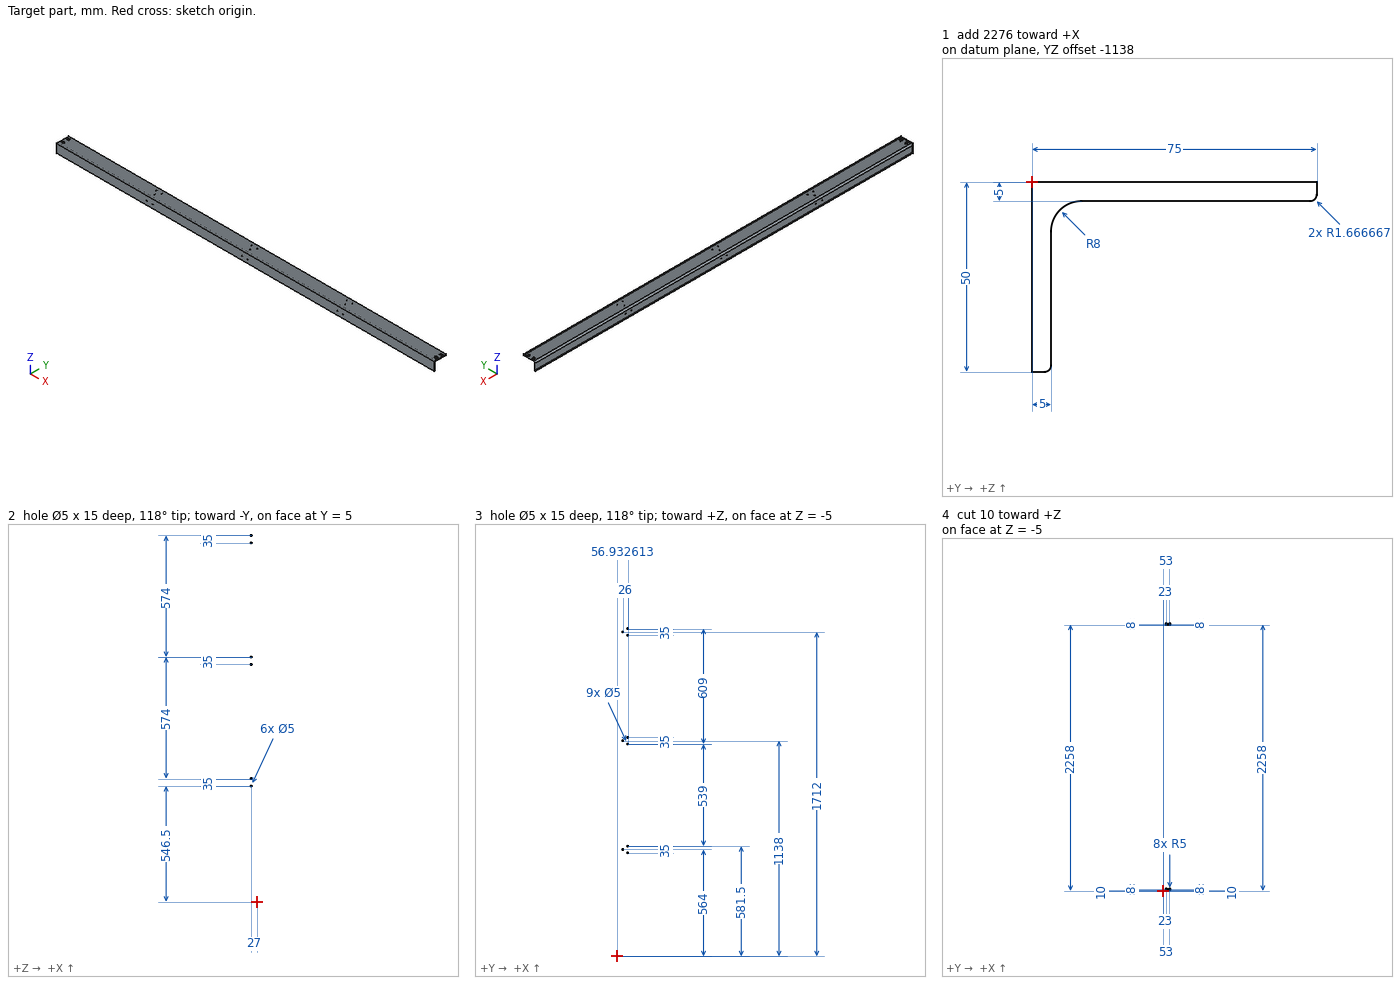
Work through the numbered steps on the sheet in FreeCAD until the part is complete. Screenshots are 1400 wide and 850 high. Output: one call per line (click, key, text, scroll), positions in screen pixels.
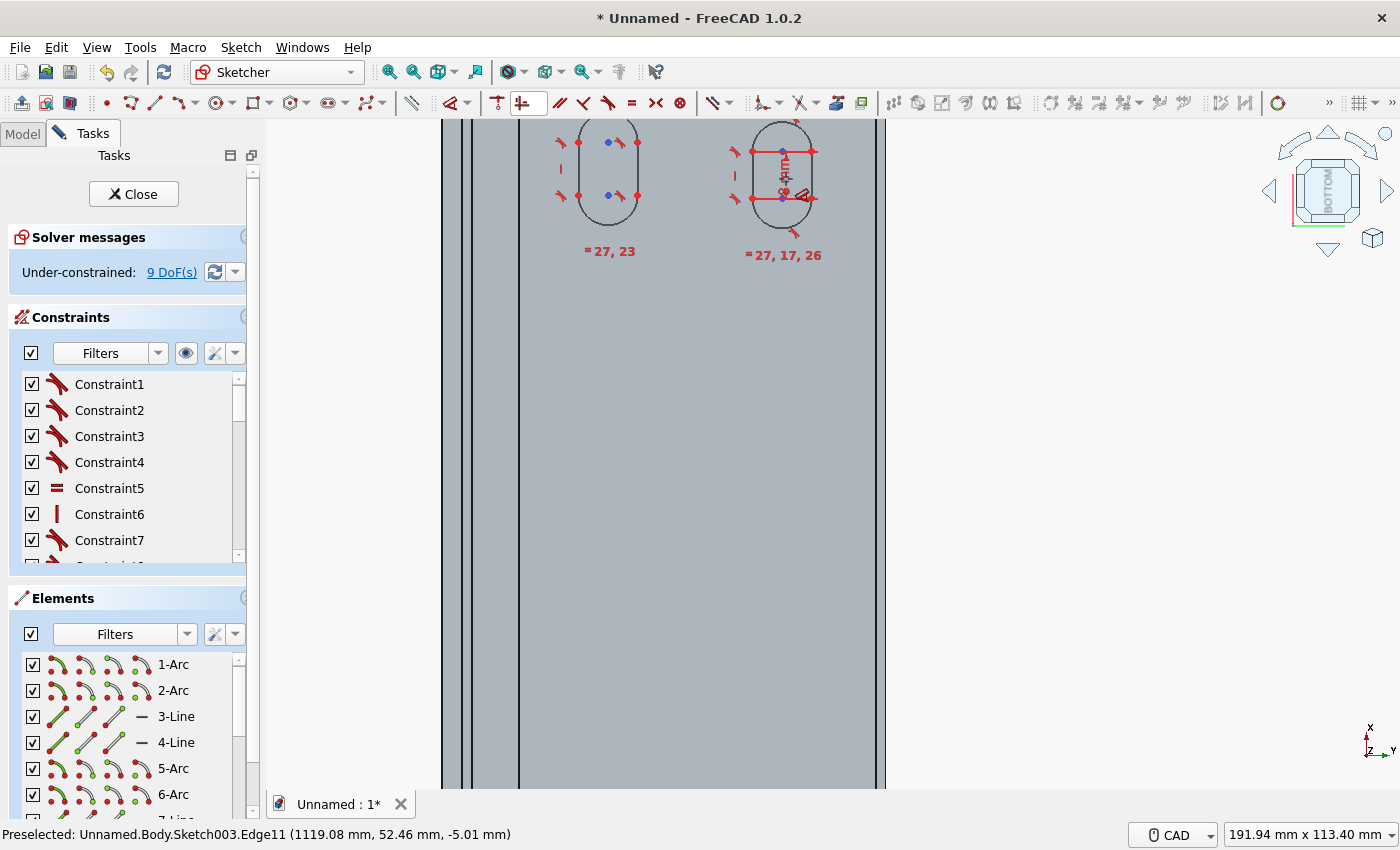
click(579, 179)
click(545, 171)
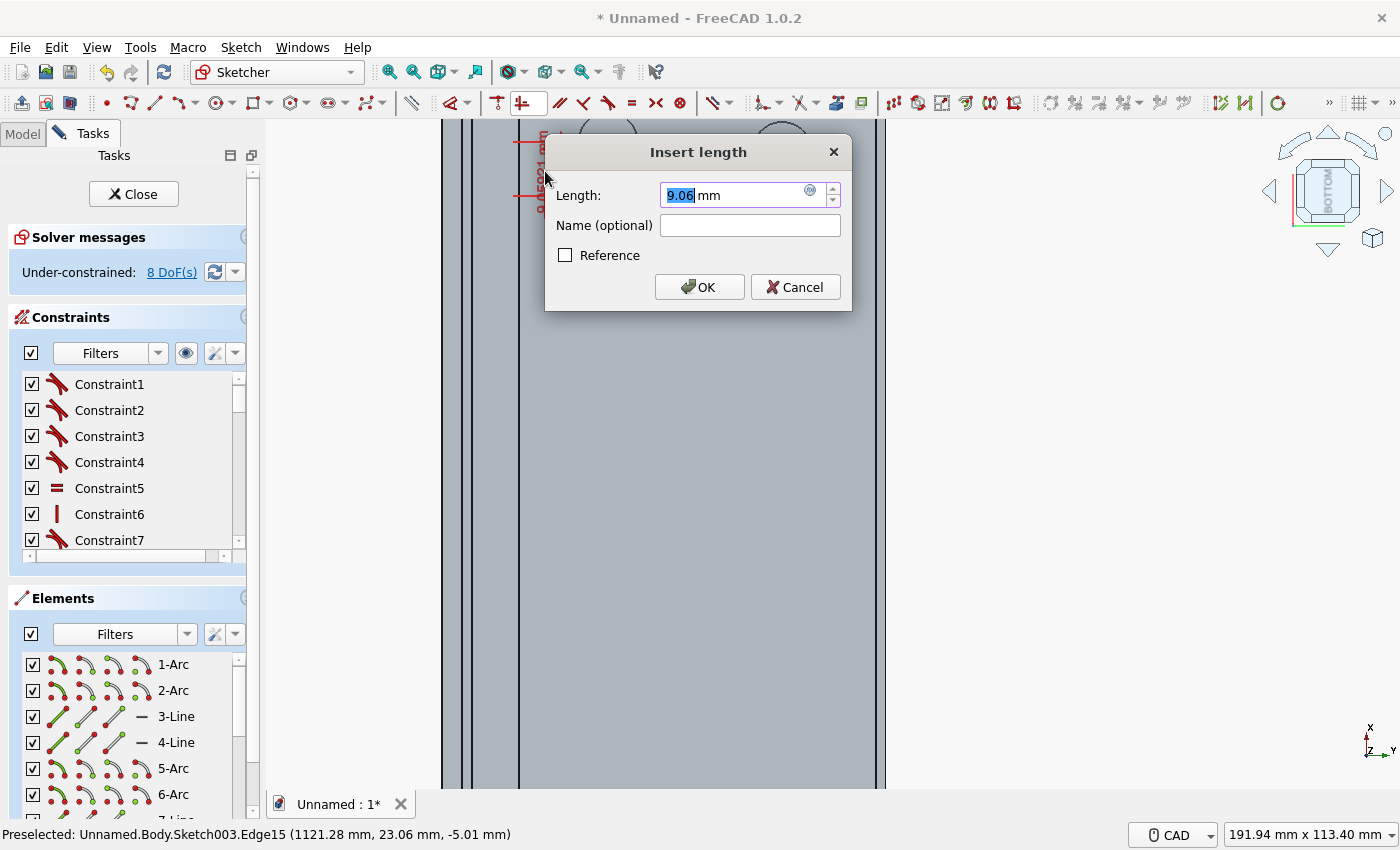
text(8)
key(Return)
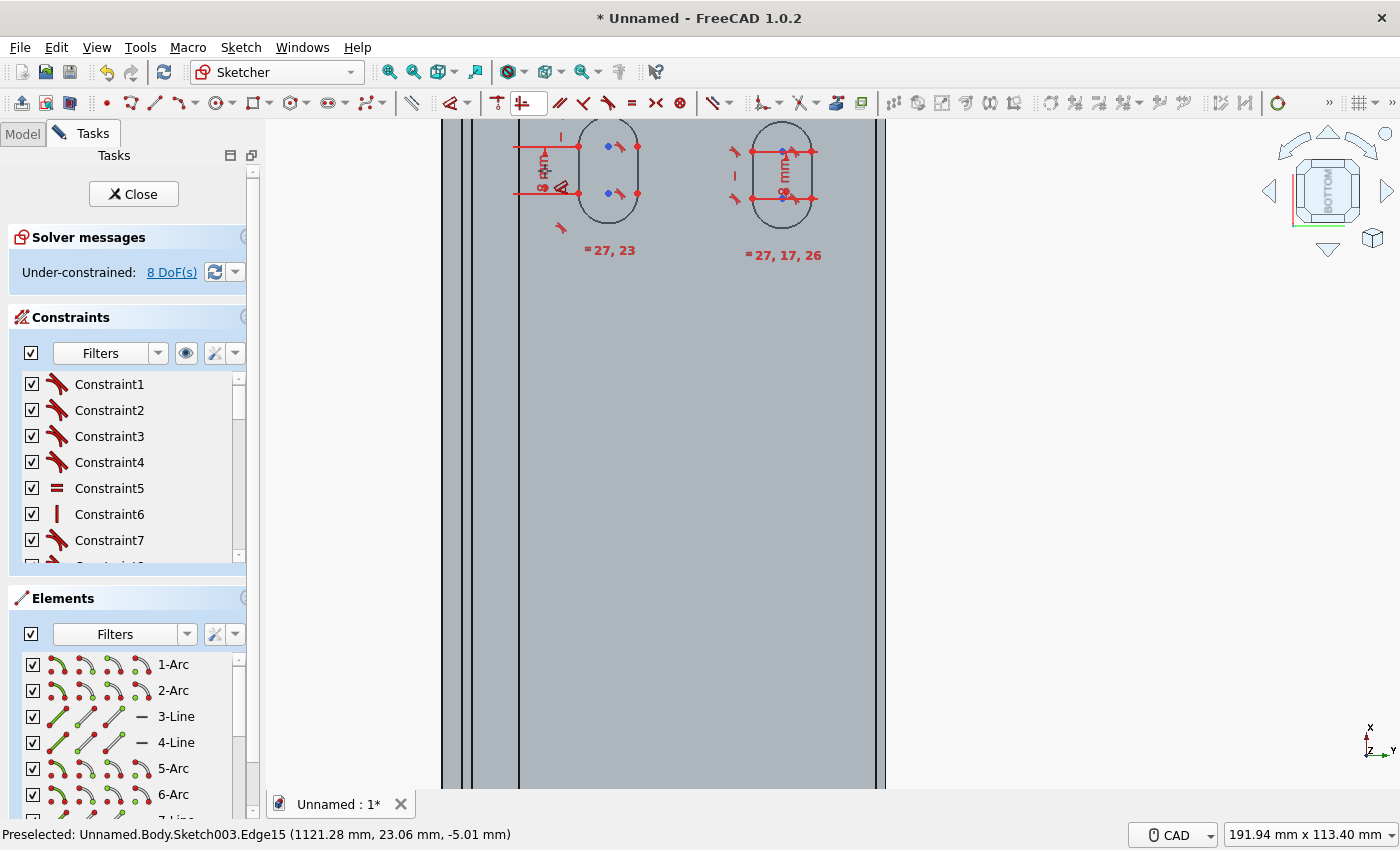
scroll(770, 184, down, 16)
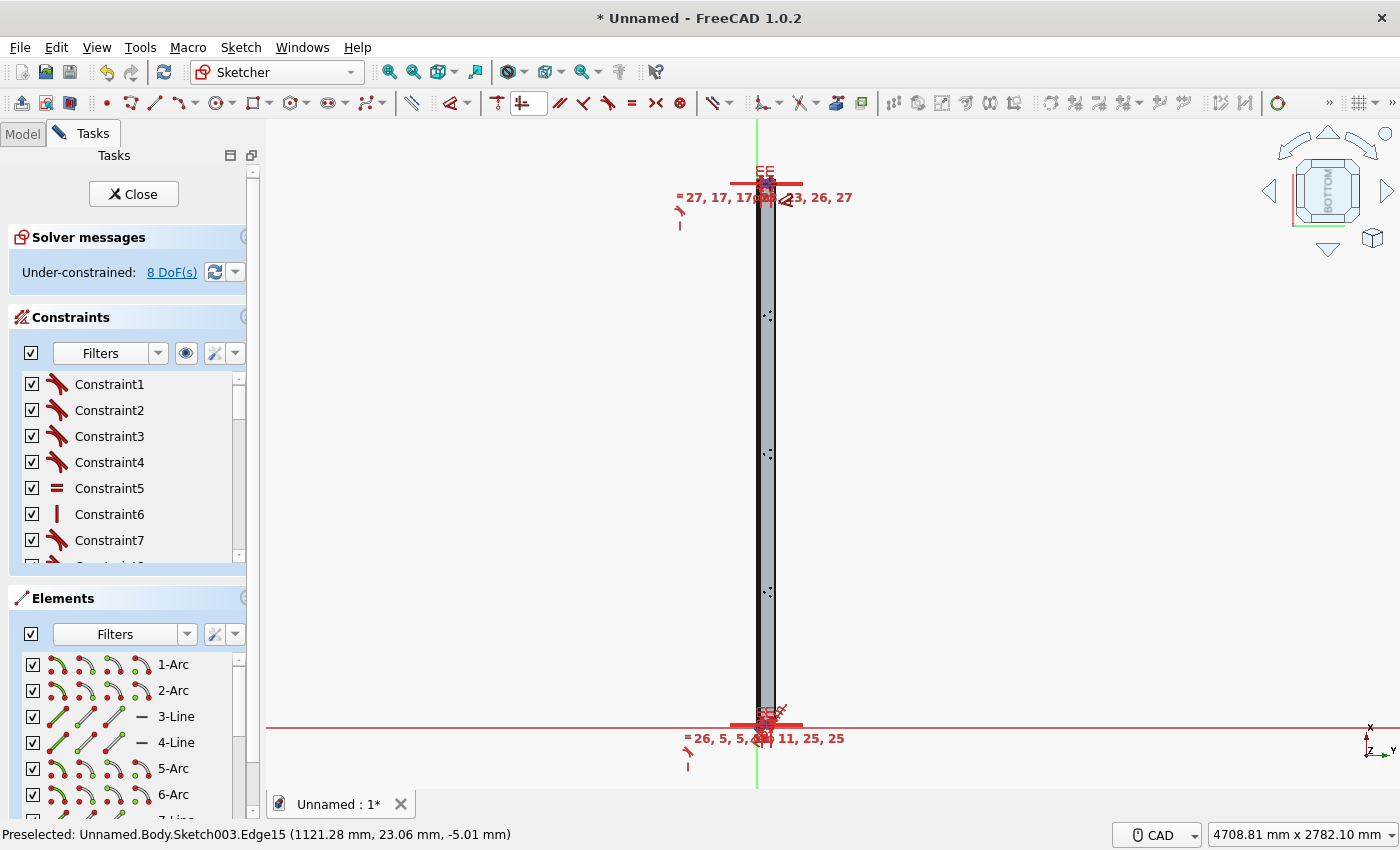
scroll(770, 726, up, 12)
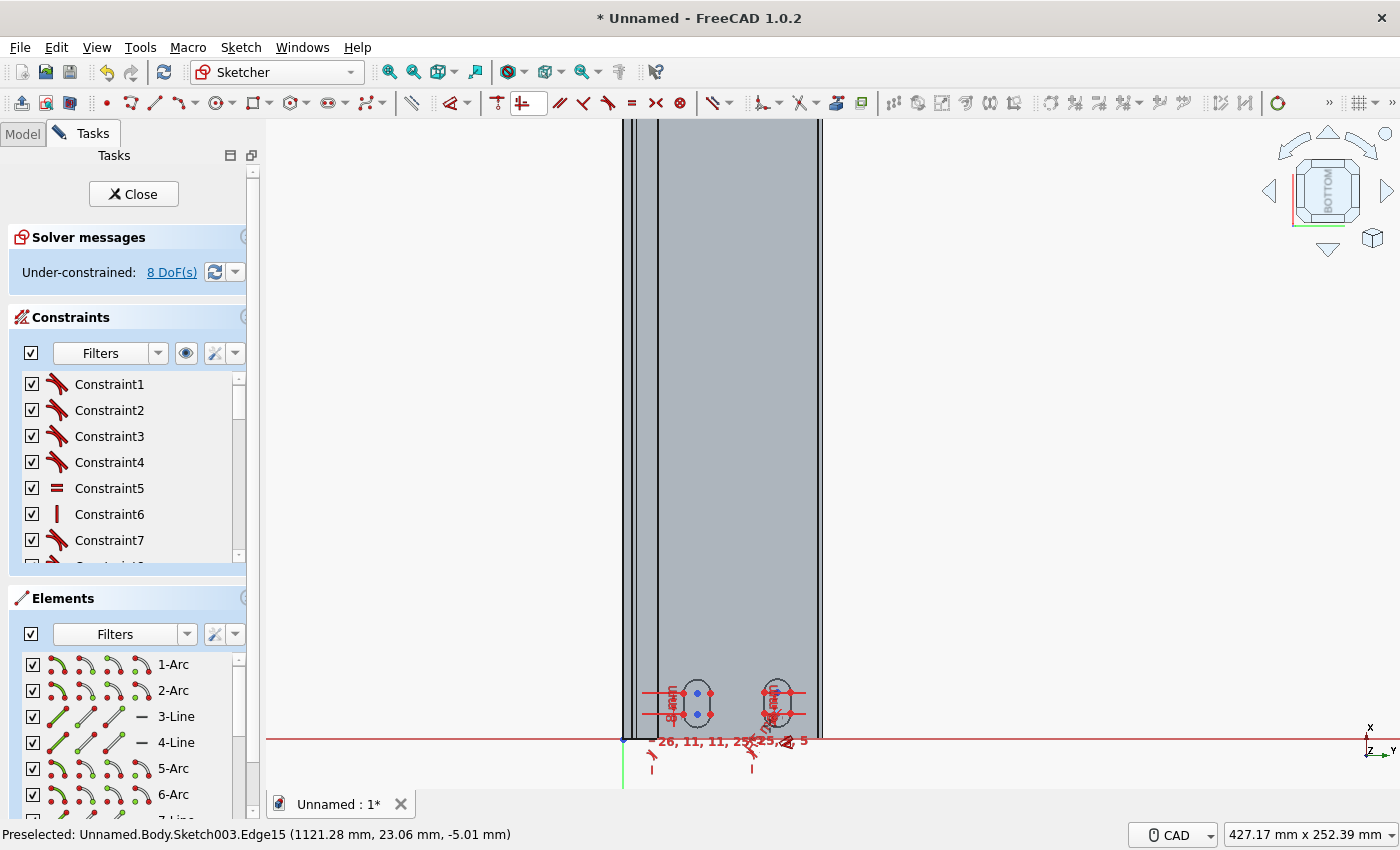
click(764, 714)
click(661, 680)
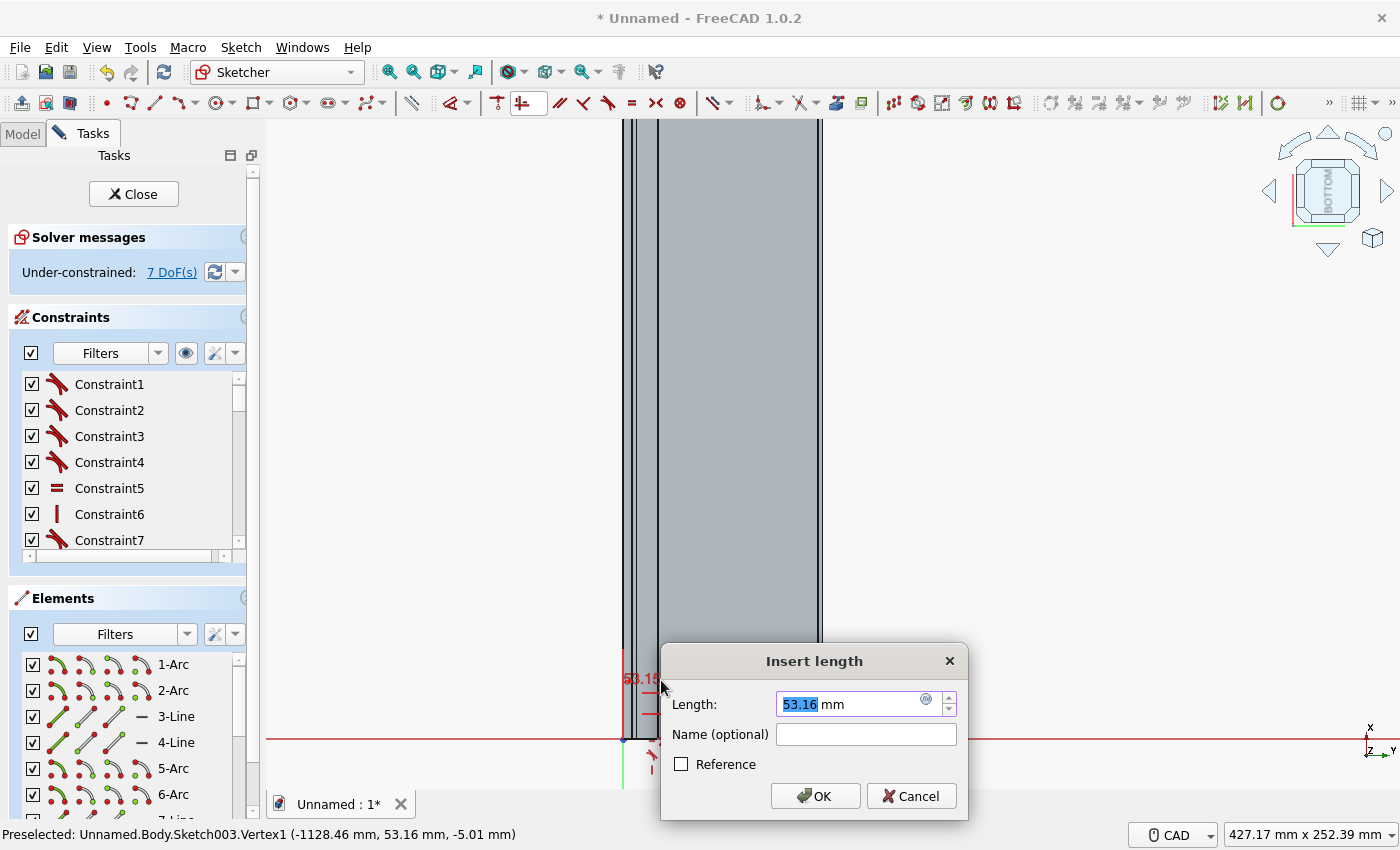
text(53)
key(Return)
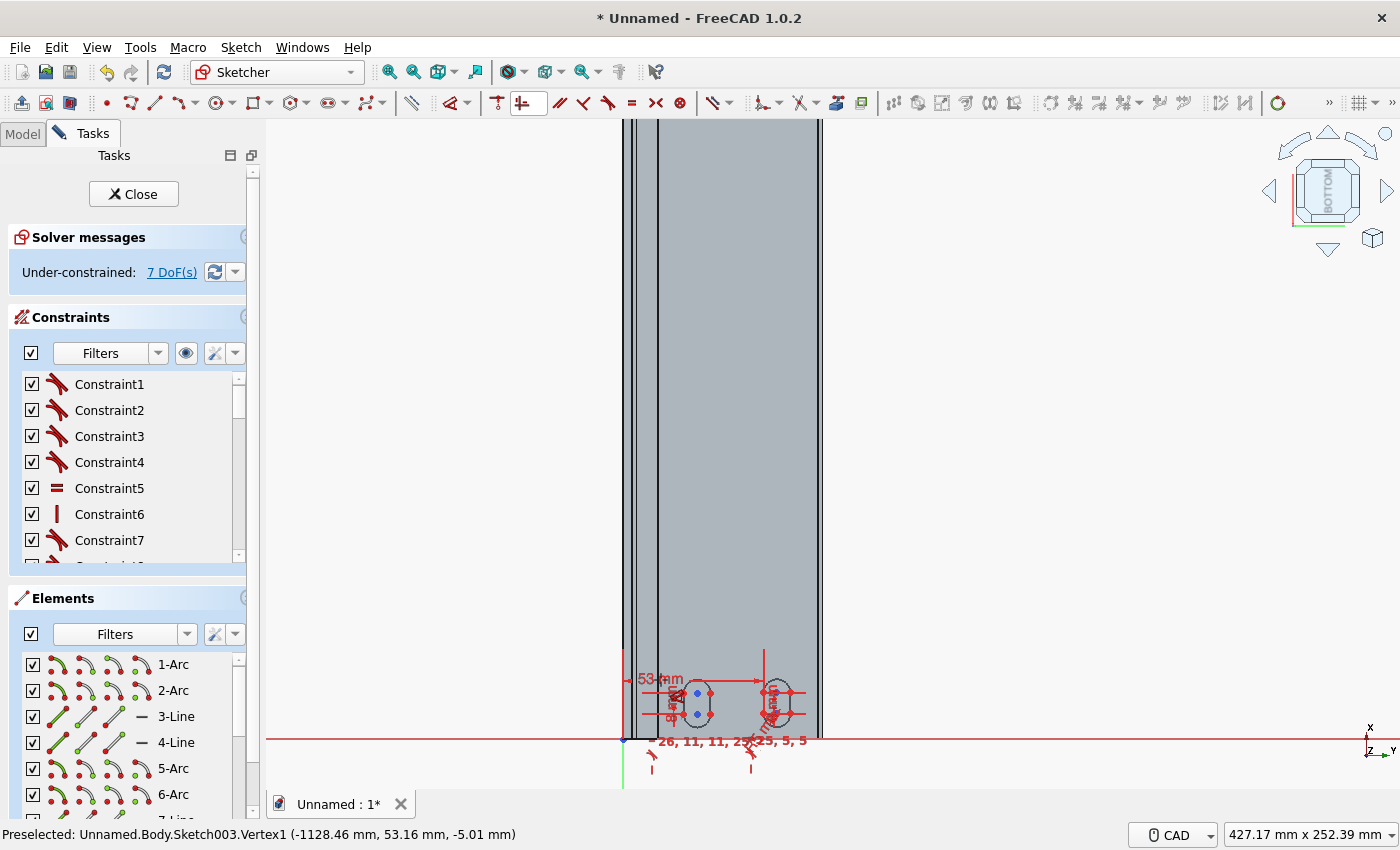
scroll(764, 714, up, 3)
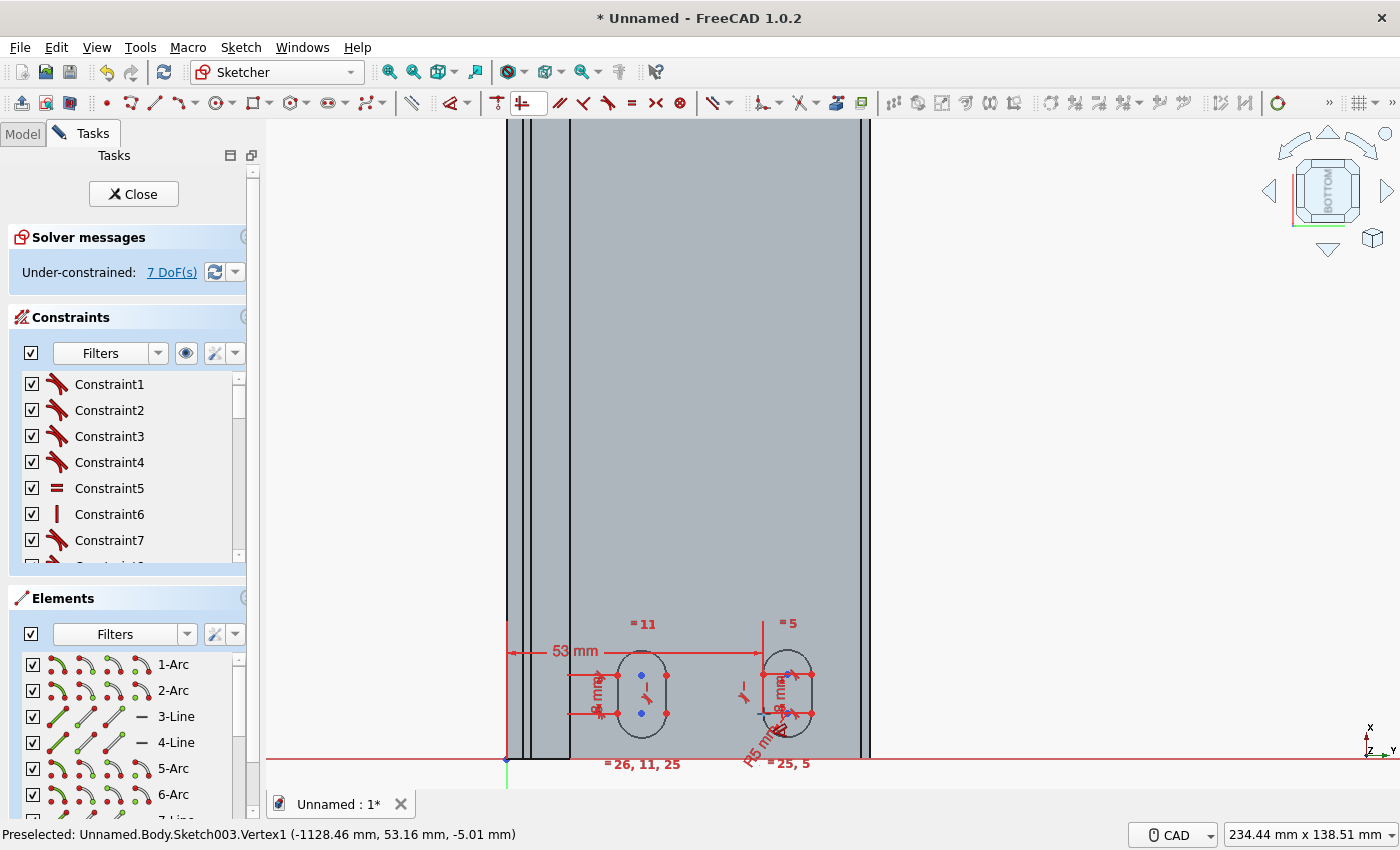
click(763, 713)
click(473, 736)